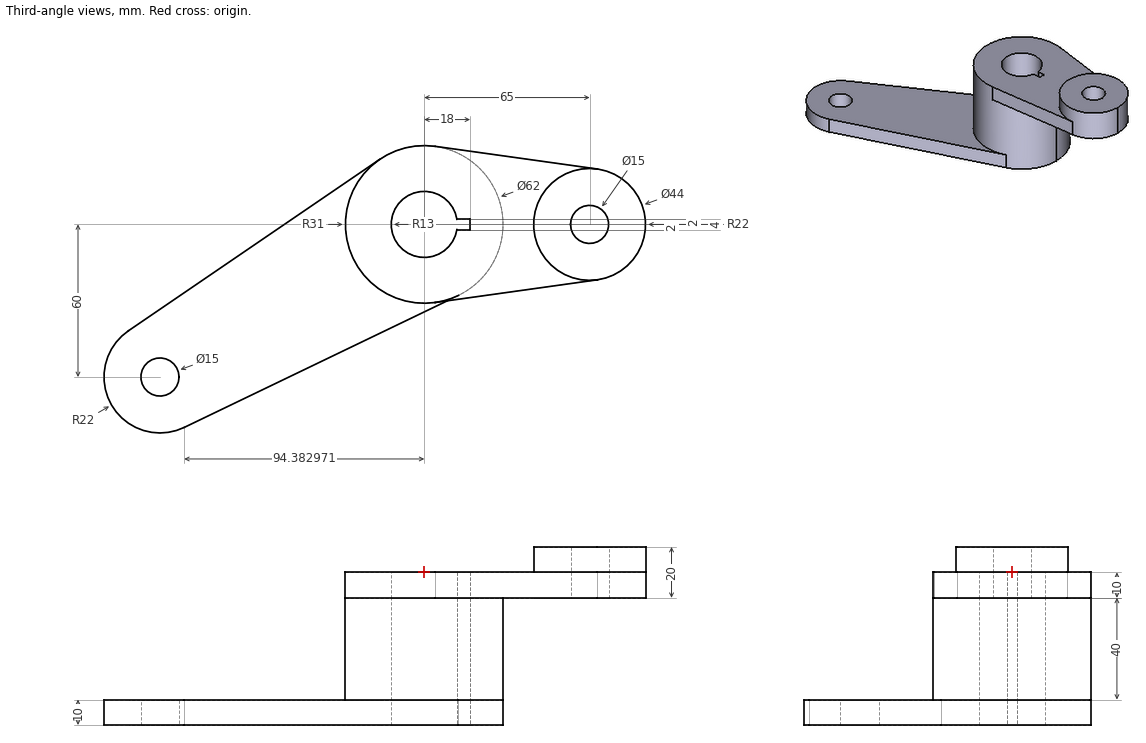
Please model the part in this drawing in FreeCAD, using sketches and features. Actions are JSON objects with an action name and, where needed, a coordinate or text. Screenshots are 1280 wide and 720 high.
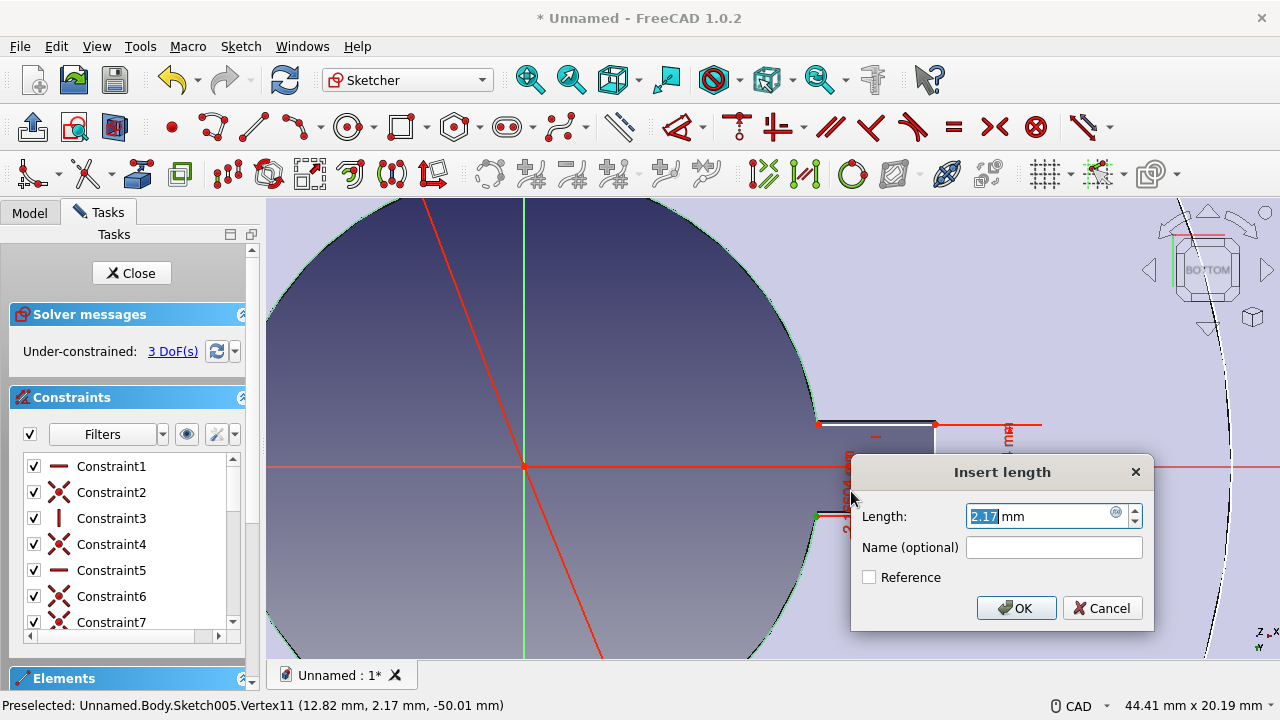
{"action": "type", "text": "2"}
{"action": "key", "text": "Return"}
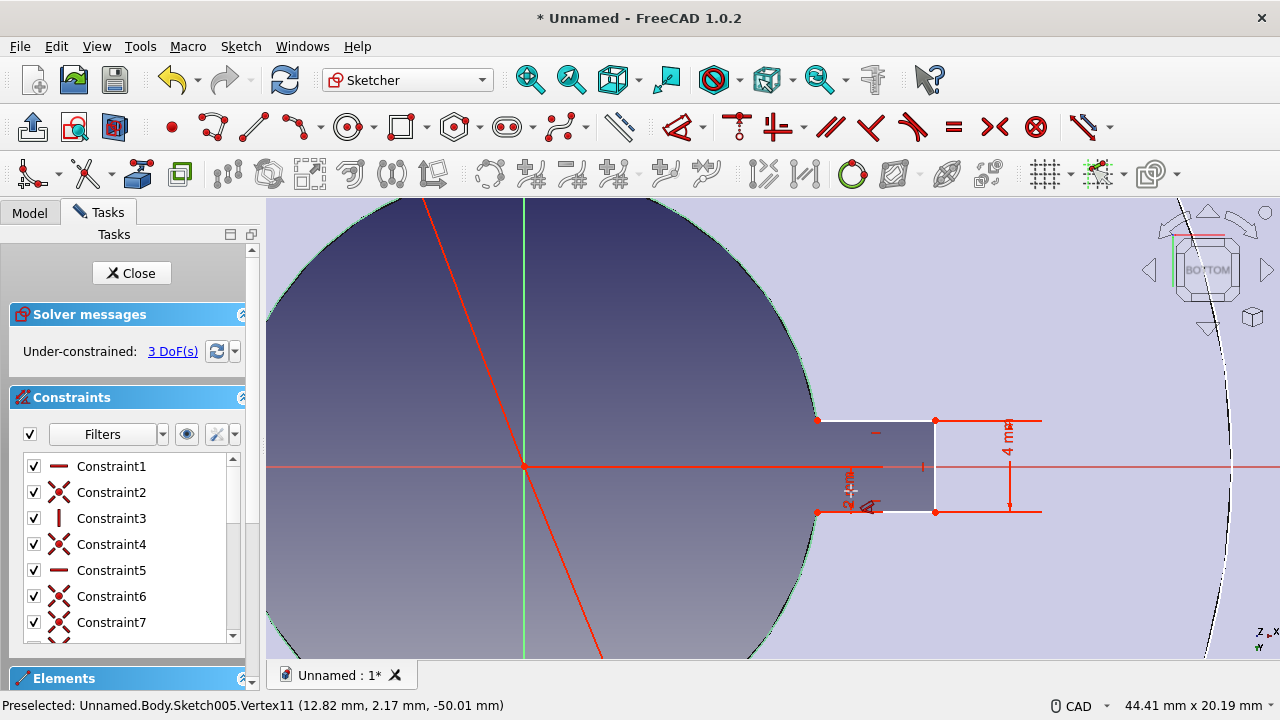
{"action": "scroll", "coordinate": [864, 501], "scroll_direction": "down", "scroll_amount": 11}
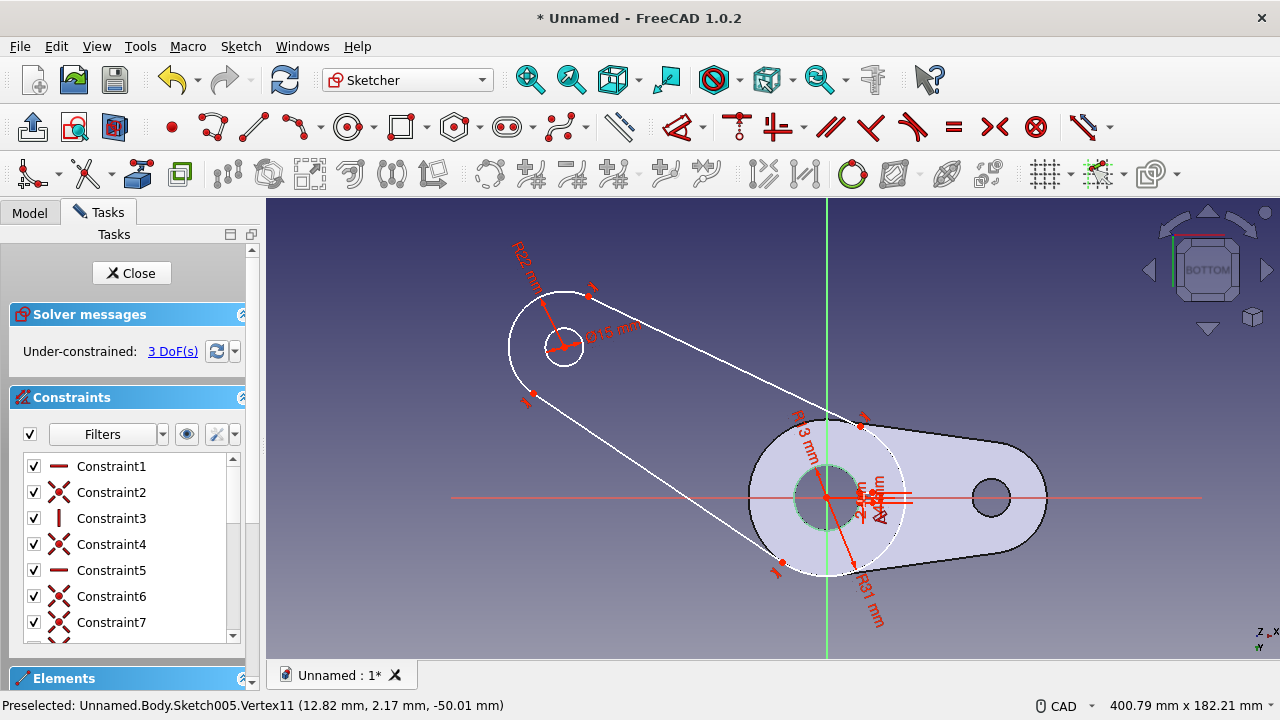
{"action": "left_click", "coordinate": [564, 347]}
{"action": "left_click", "coordinate": [530, 422]}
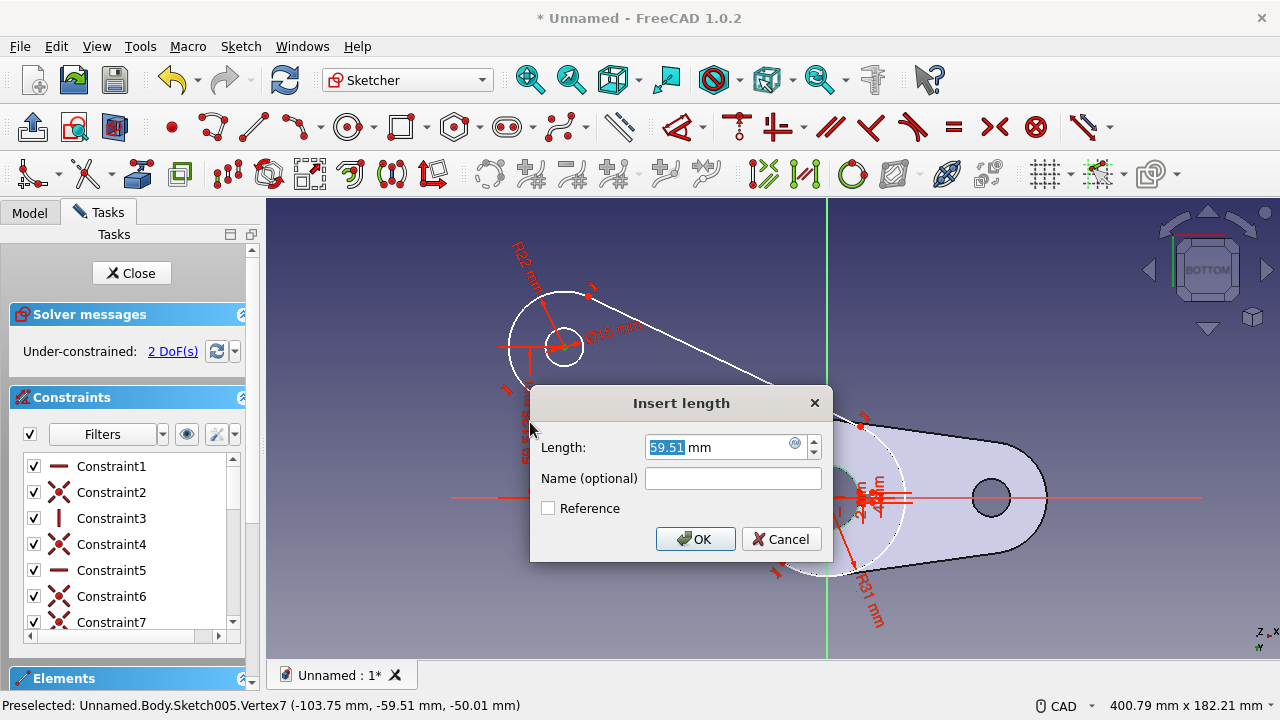
{"action": "type", "text": "60"}
{"action": "key", "text": "Return"}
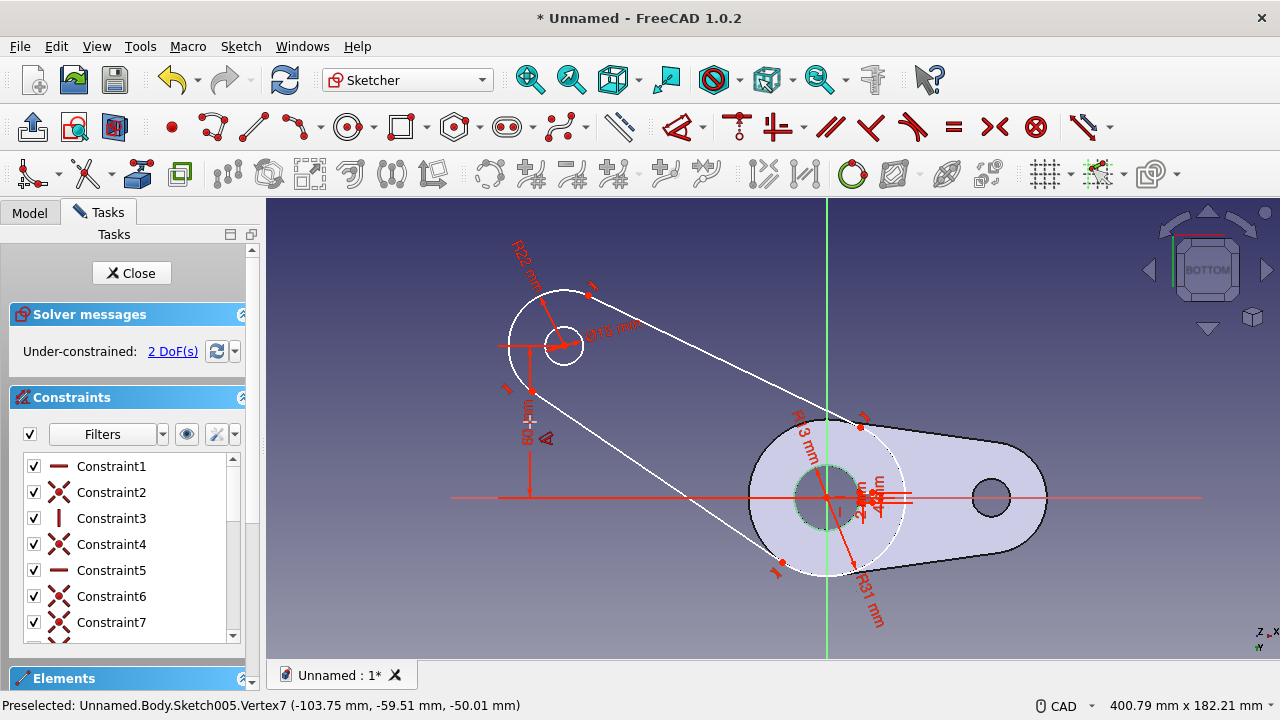
{"action": "left_click", "coordinate": [872, 503]}
{"action": "left_click", "coordinate": [860, 537]}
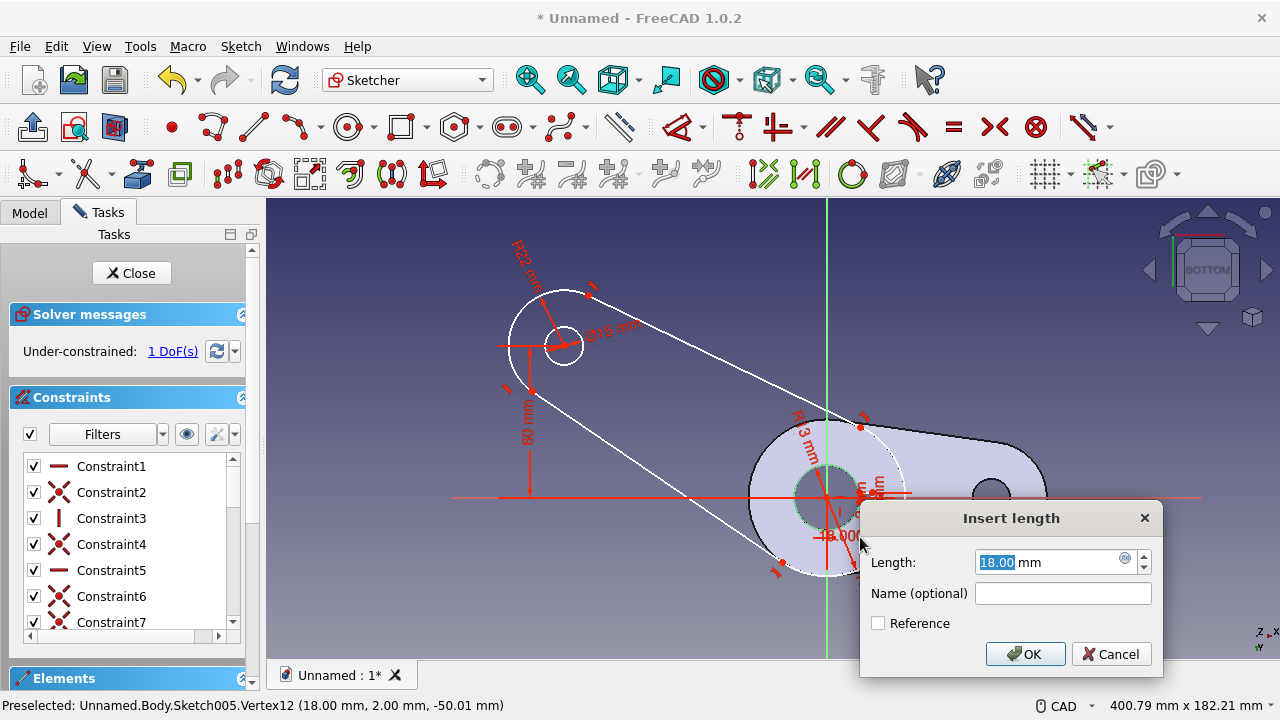
{"action": "type", "text": "18"}
{"action": "key", "text": "Return"}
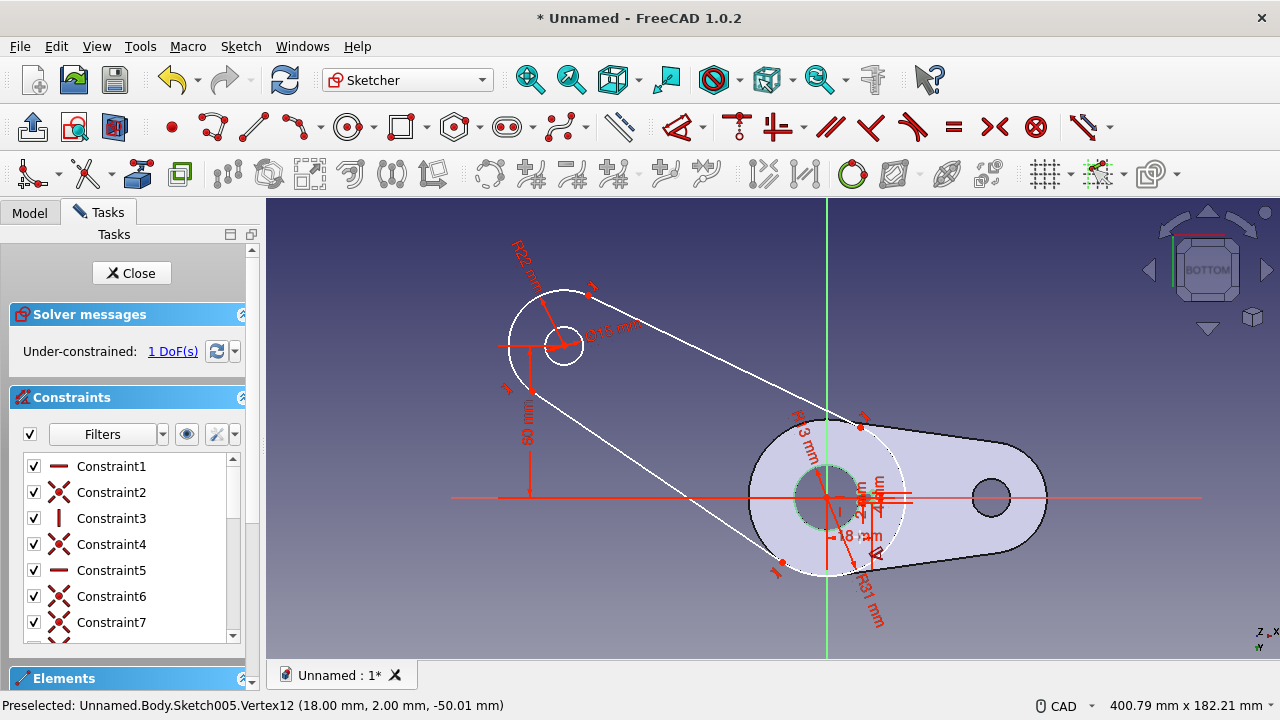
{"action": "left_click", "coordinate": [588, 296]}
{"action": "left_click", "coordinate": [708, 262]}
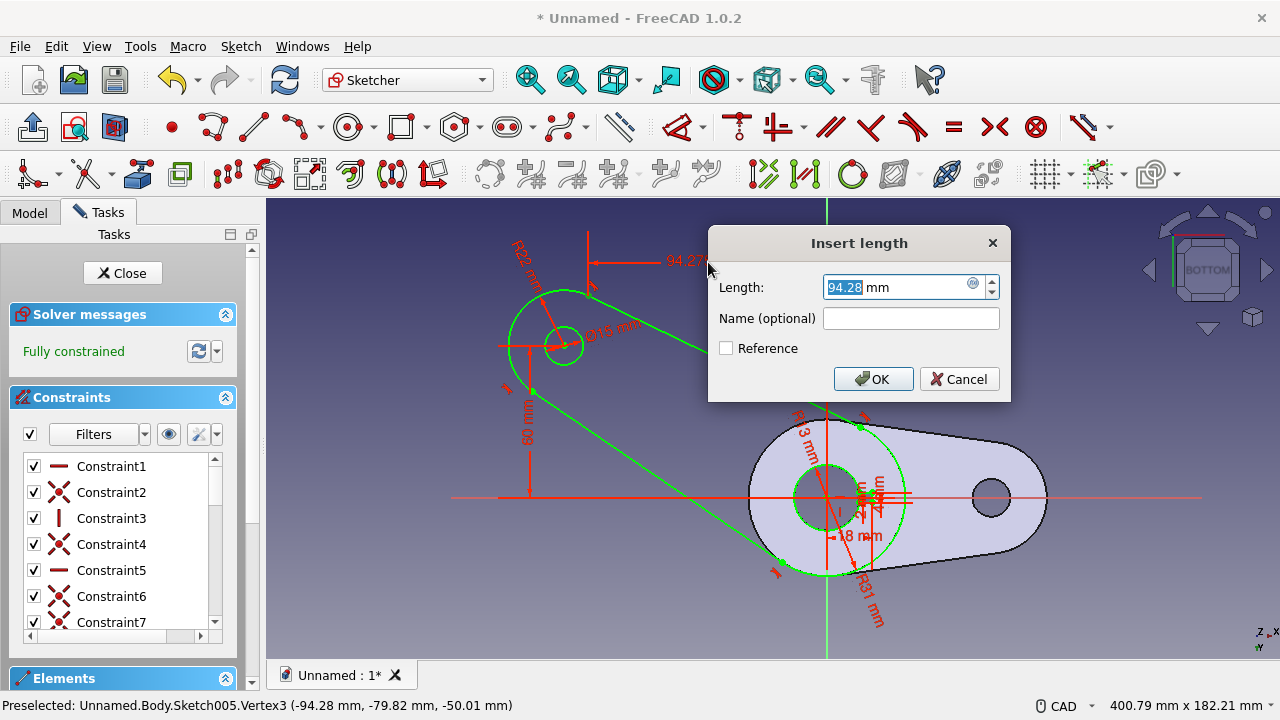
{"action": "type", "text": "94.382971"}
{"action": "key", "text": "Return"}
{"action": "key", "text": "Escape"}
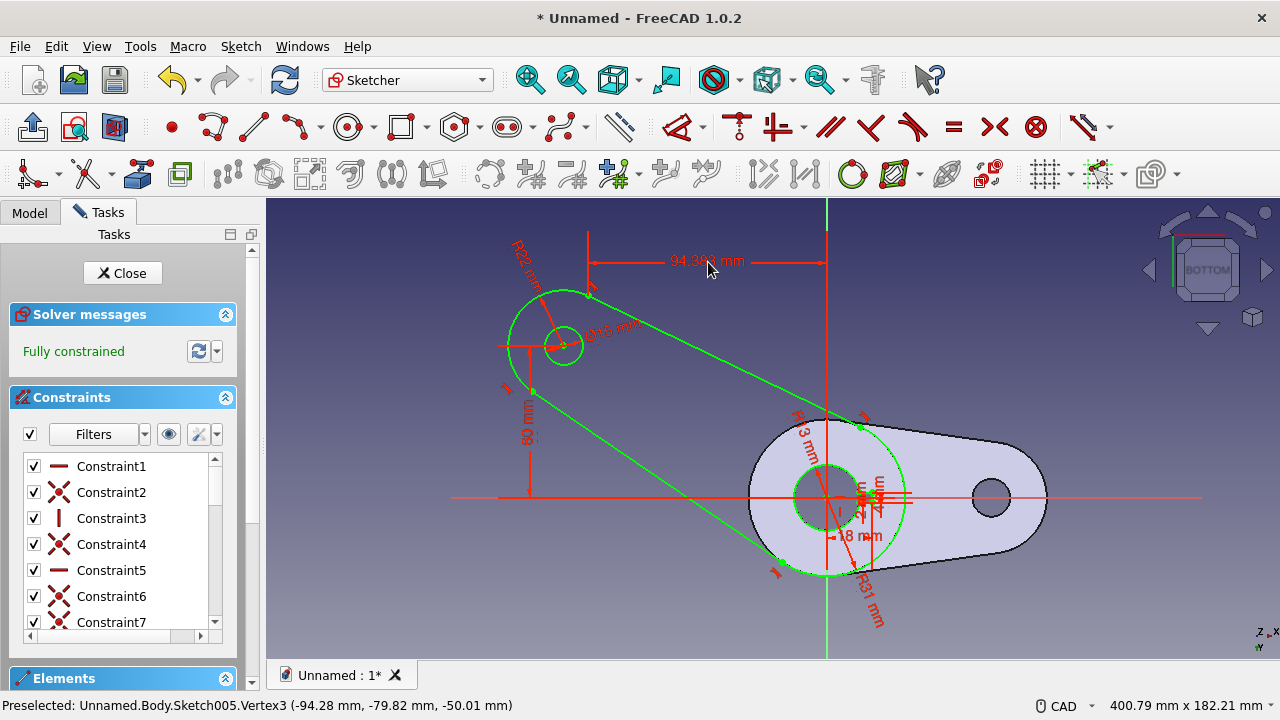
{"action": "left_click", "coordinate": [123, 273]}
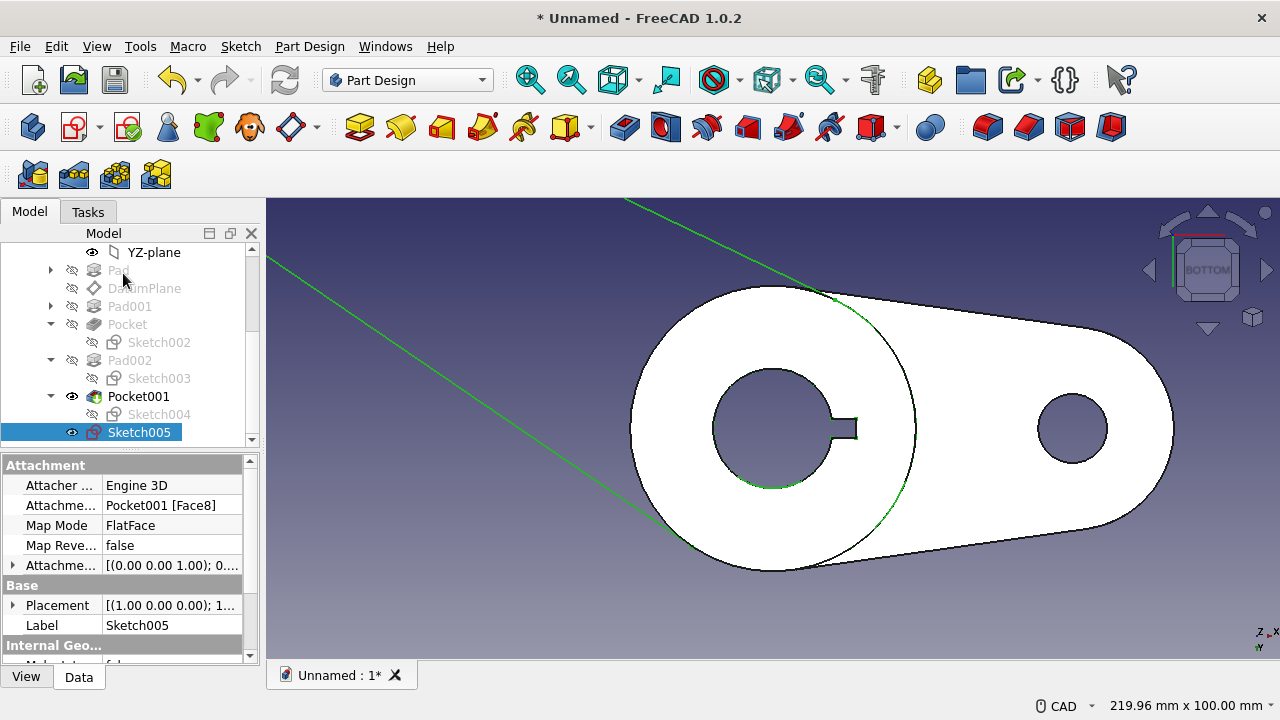
{"action": "left_click", "coordinate": [360, 128]}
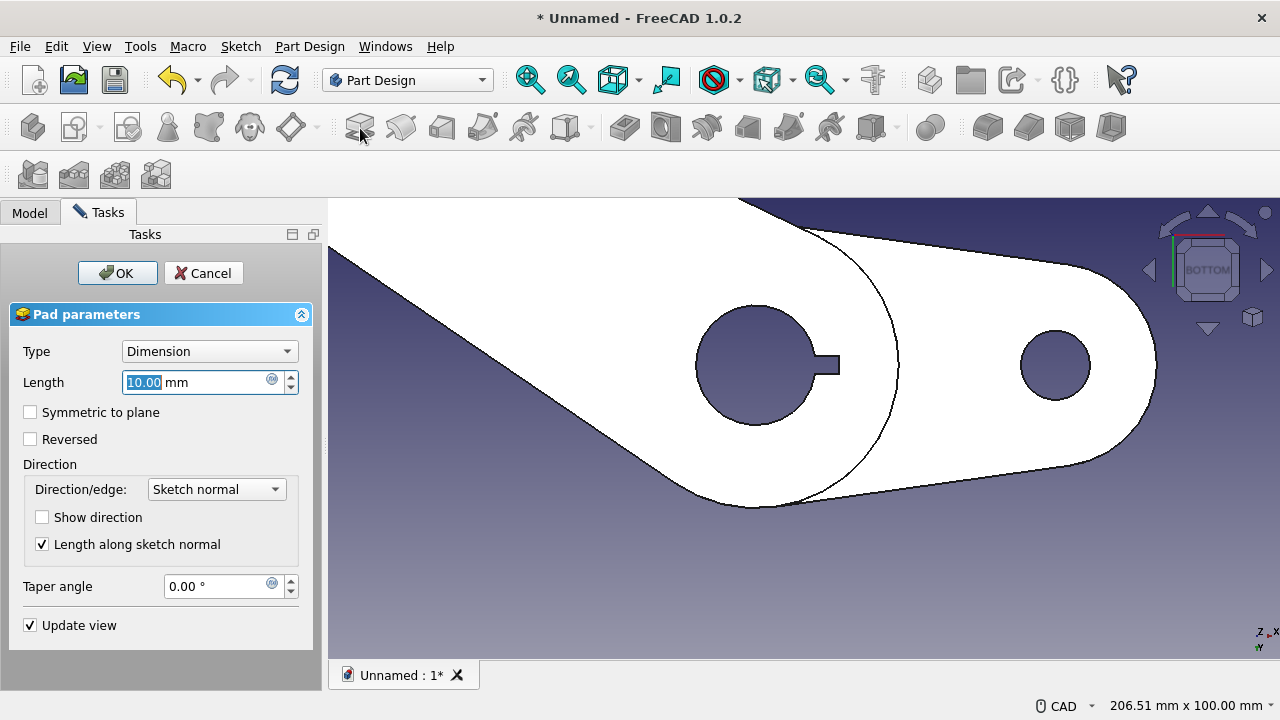
{"action": "type", "text": "10"}
{"action": "key", "text": "Tab"}